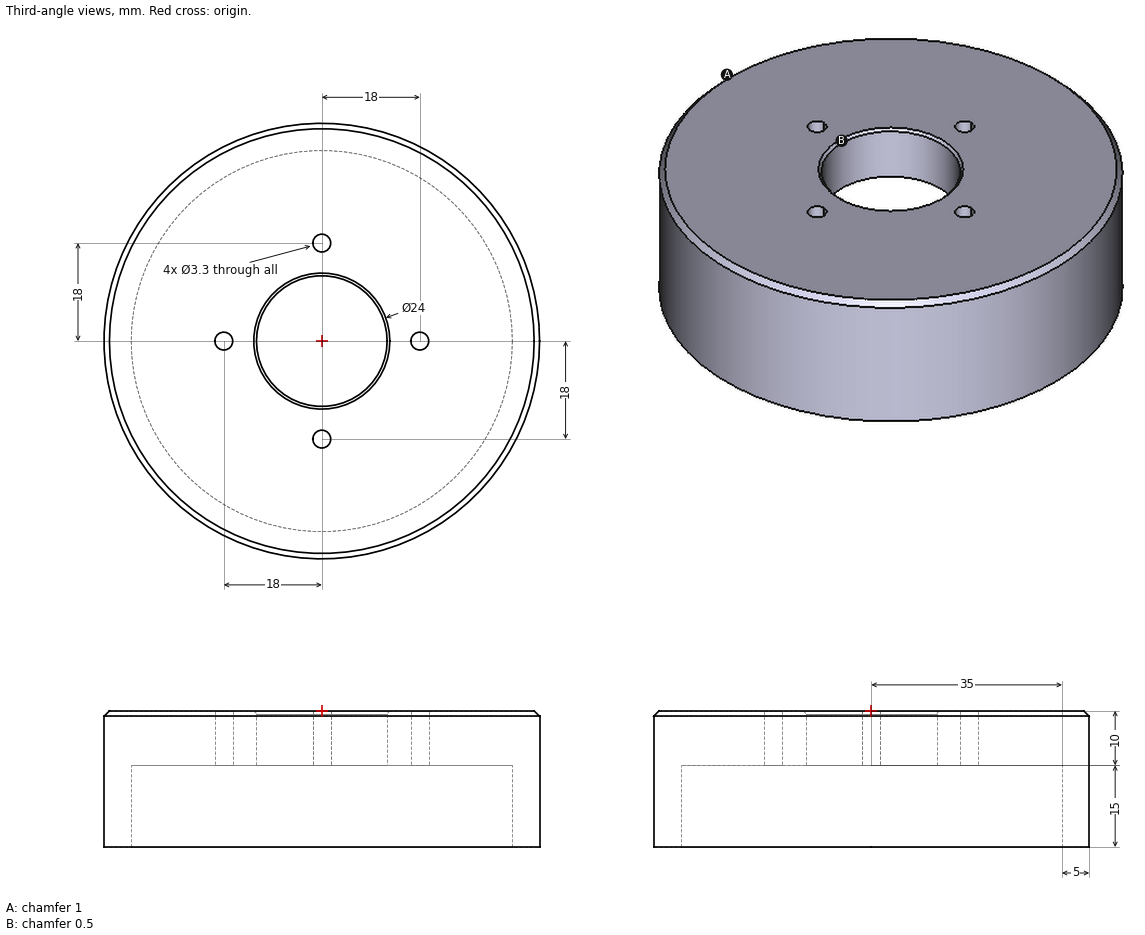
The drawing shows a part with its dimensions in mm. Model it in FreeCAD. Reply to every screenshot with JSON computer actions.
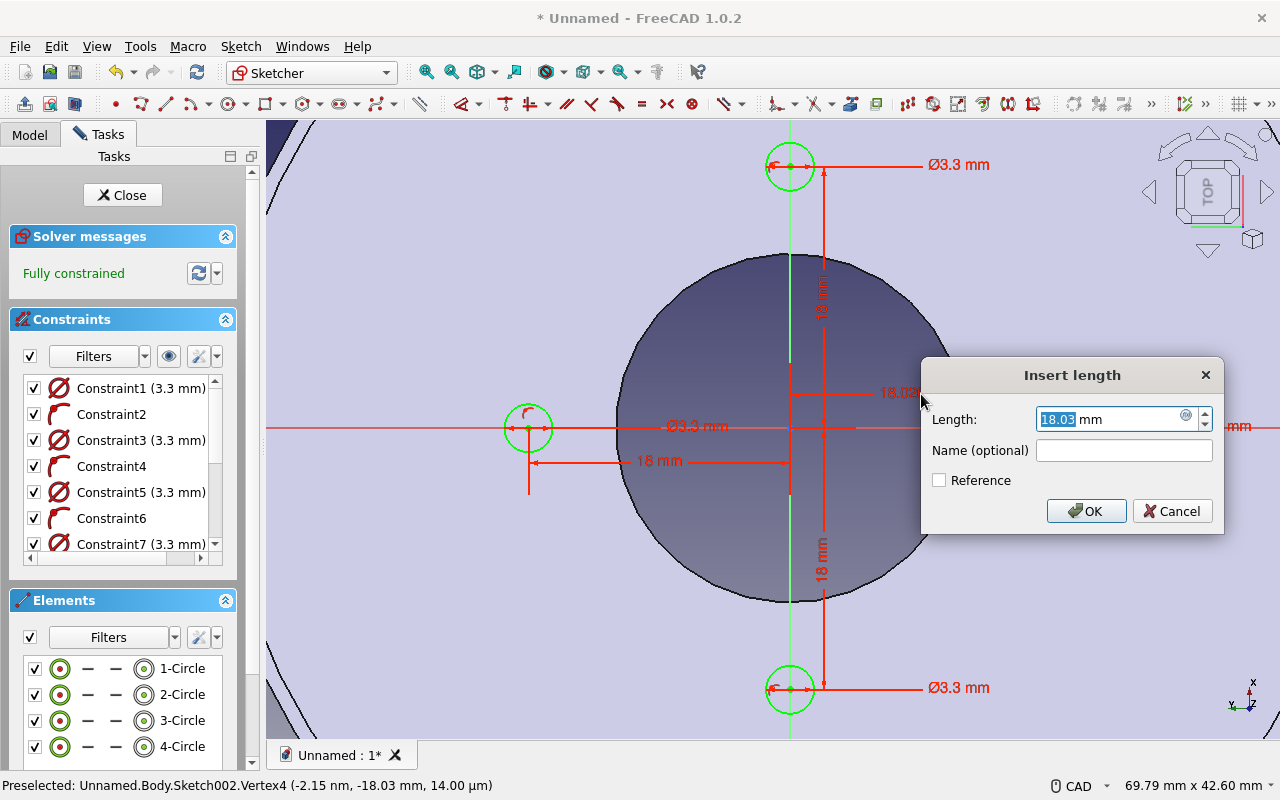
{"action": "type", "text": "18"}
{"action": "key", "text": "Return"}
{"action": "key", "text": "Escape"}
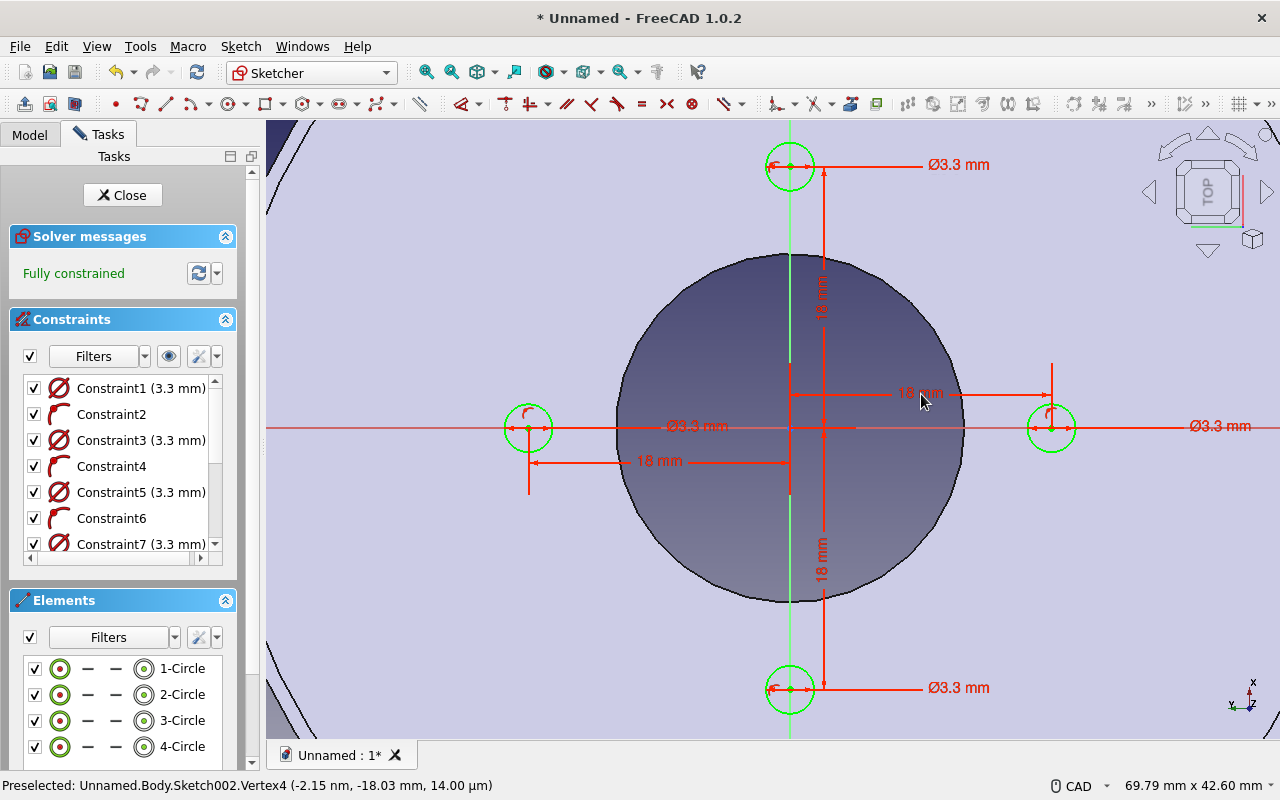
{"action": "left_click", "coordinate": [123, 195]}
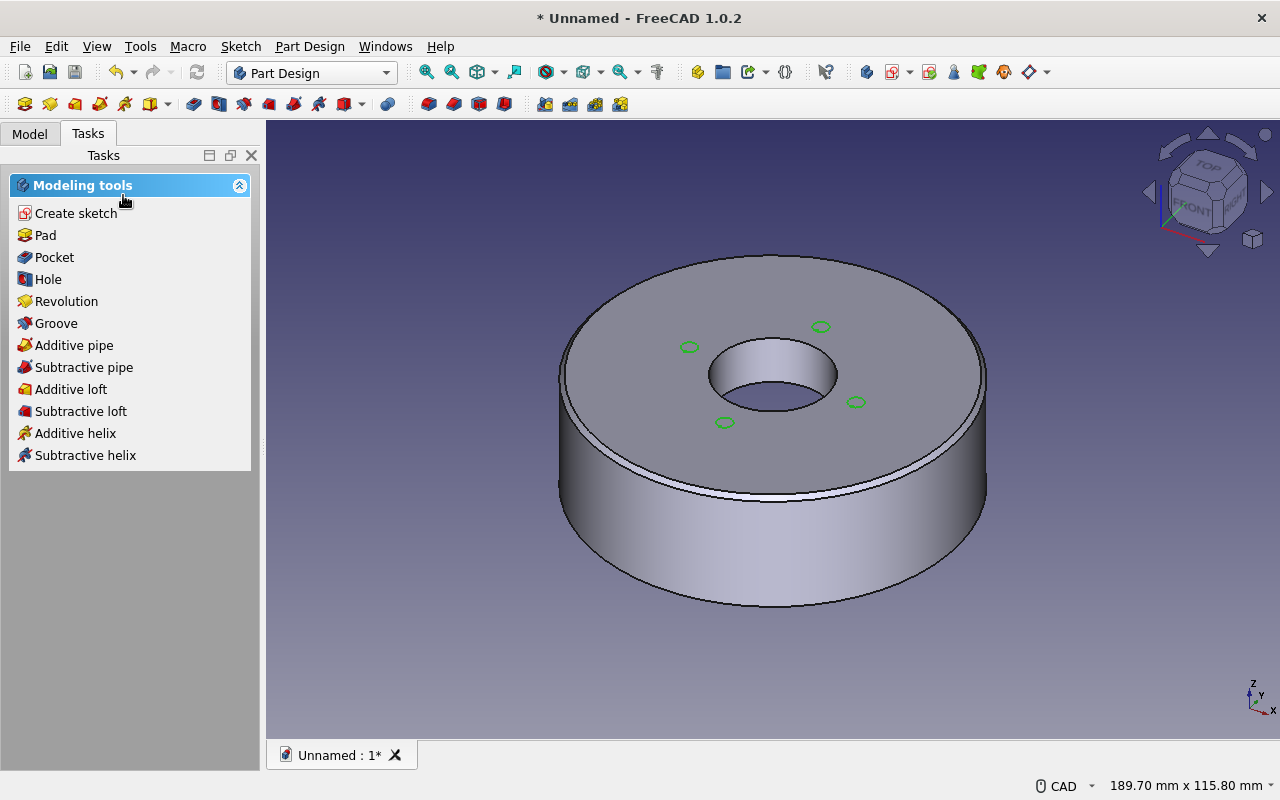
{"action": "left_click", "coordinate": [219, 104]}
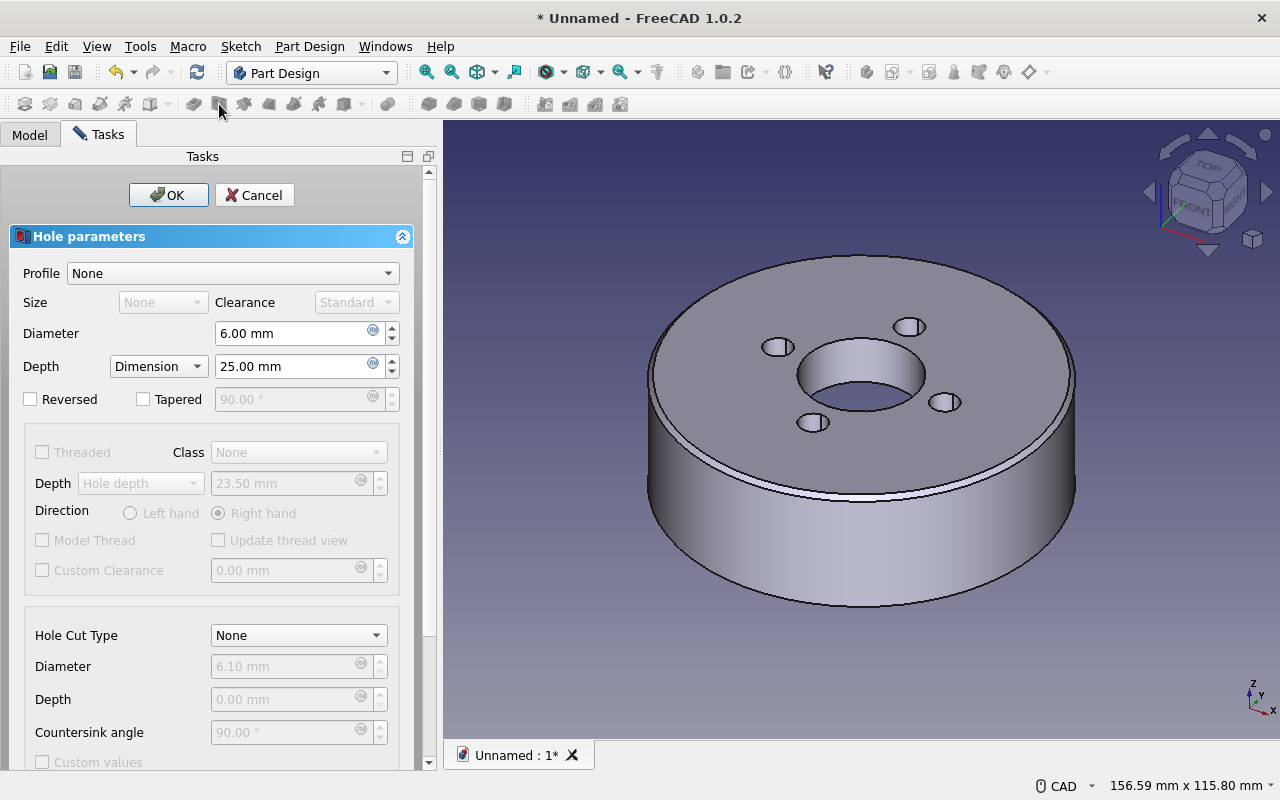
{"action": "triple_click", "coordinate": [300, 334]}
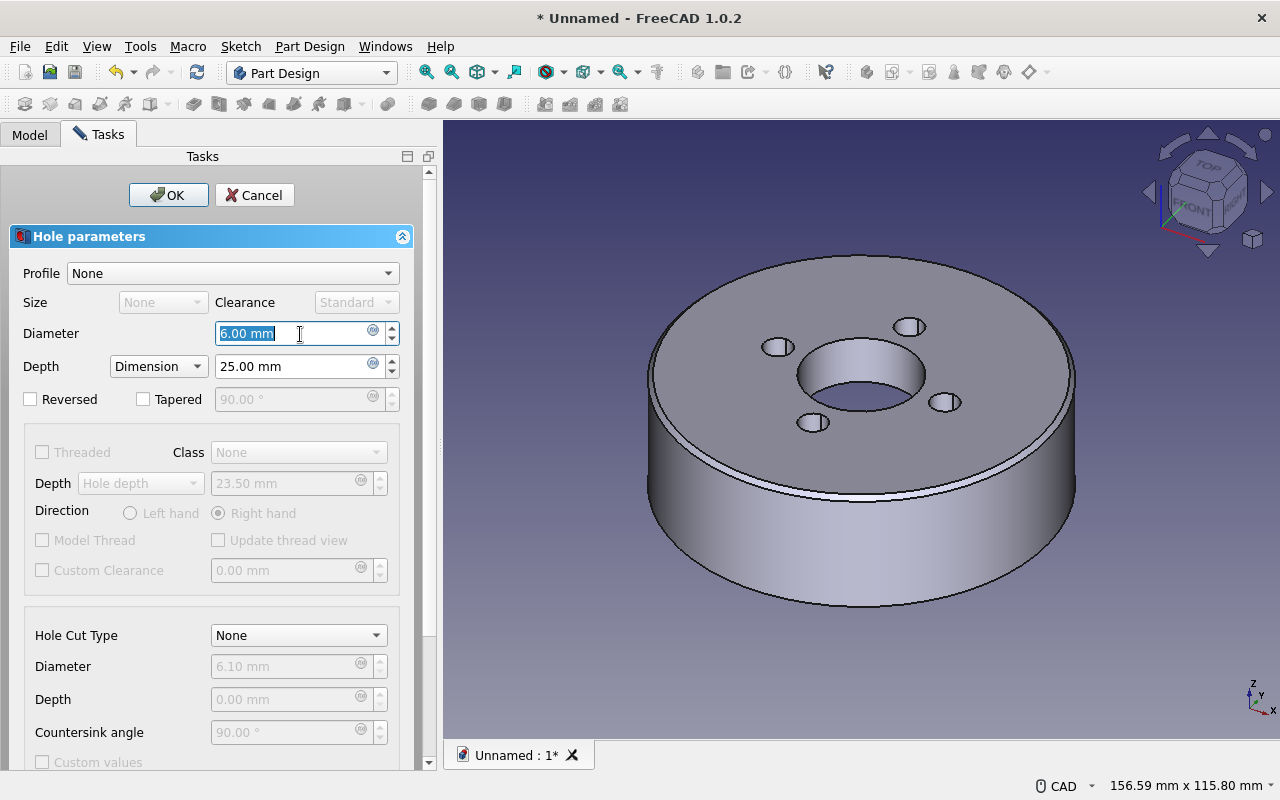
{"action": "type", "text": "3.3"}
{"action": "key", "text": "Tab"}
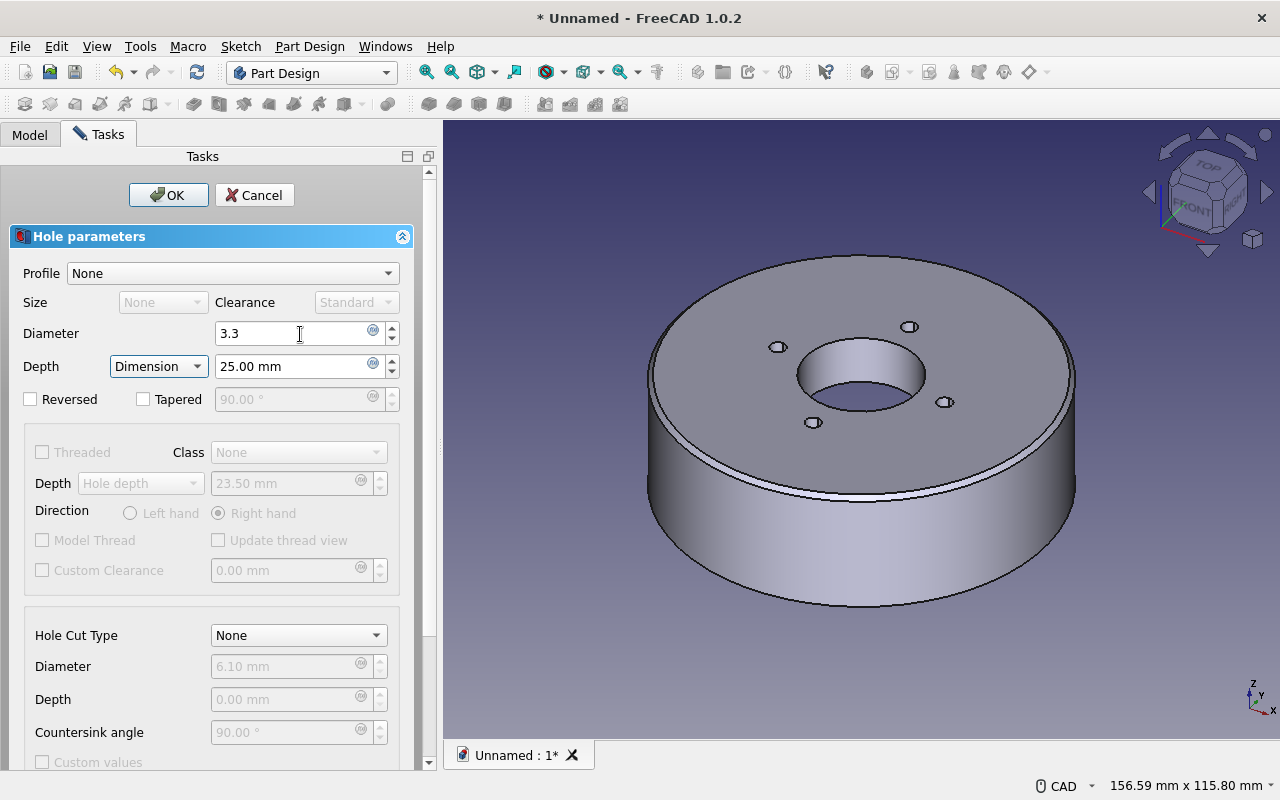
{"action": "left_click", "coordinate": [160, 366]}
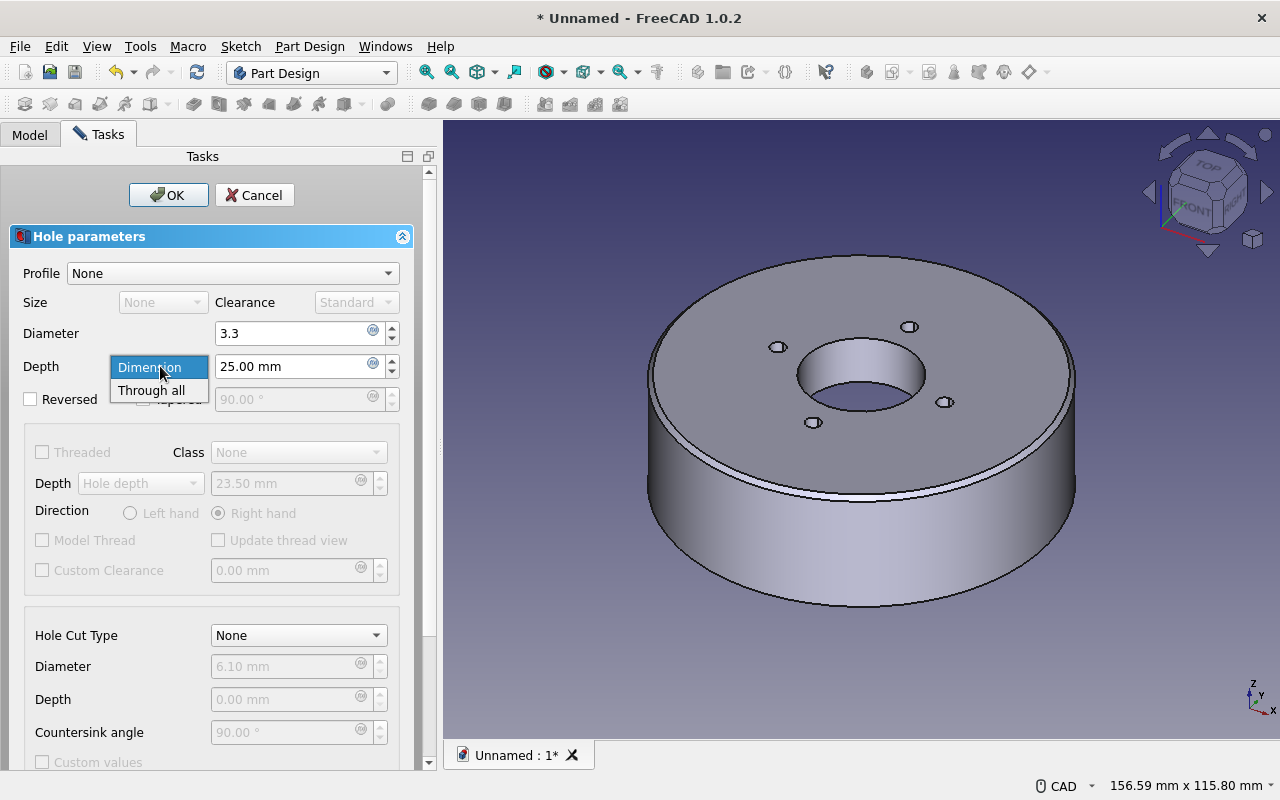
{"action": "left_click", "coordinate": [158, 390]}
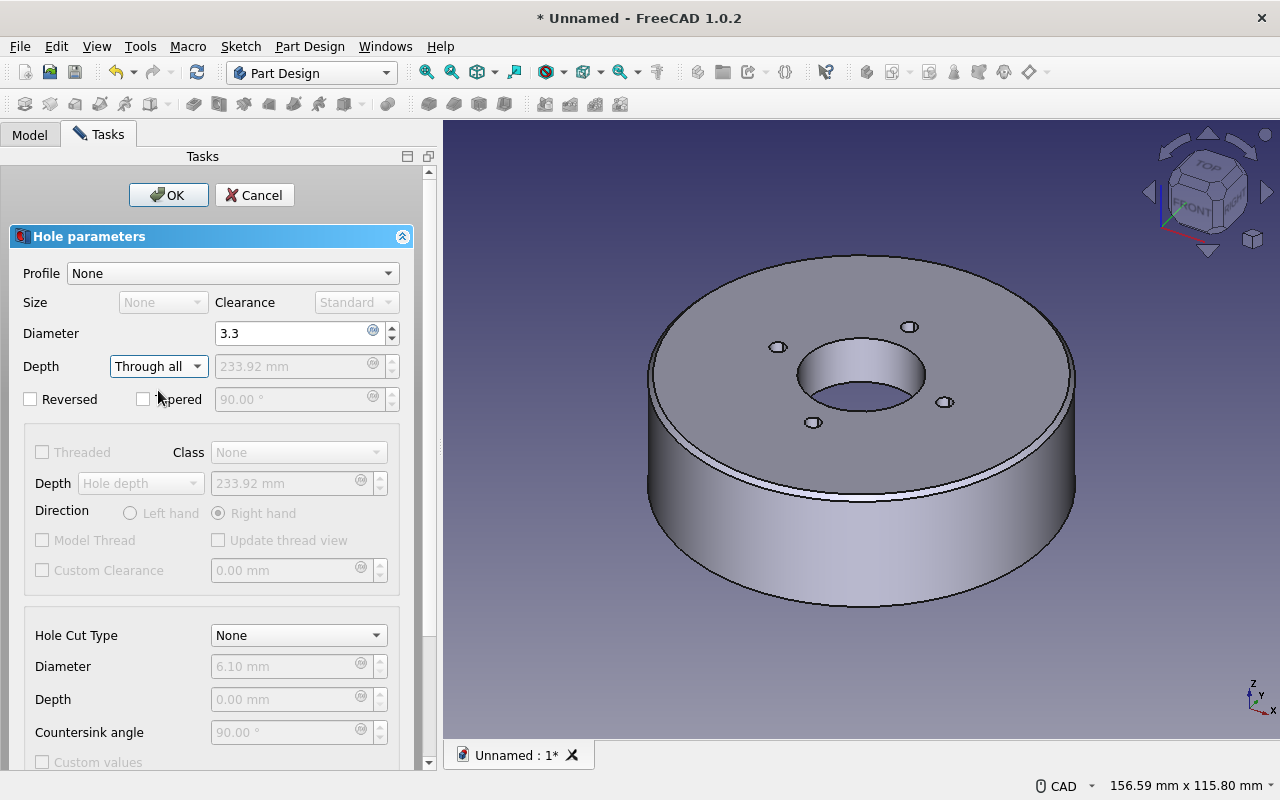
{"action": "left_click", "coordinate": [169, 195]}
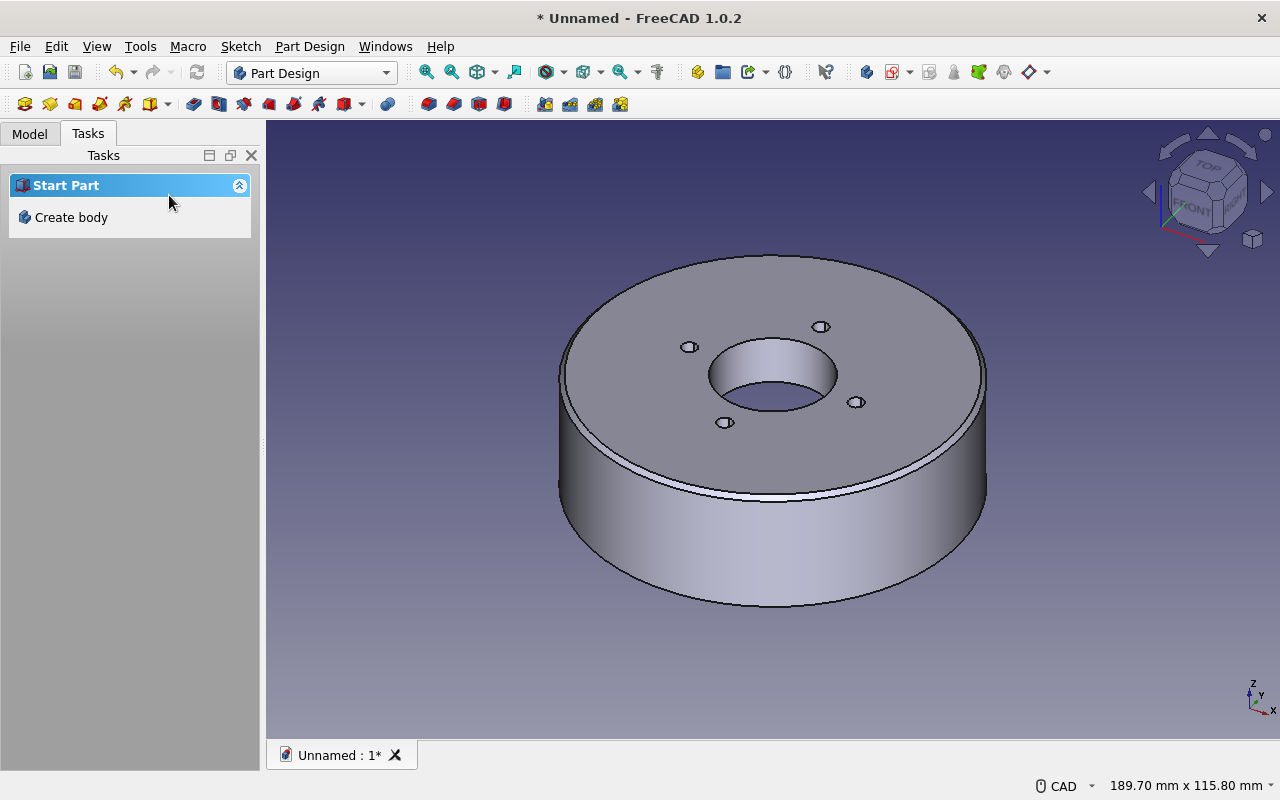
{"action": "left_click", "coordinate": [805, 342]}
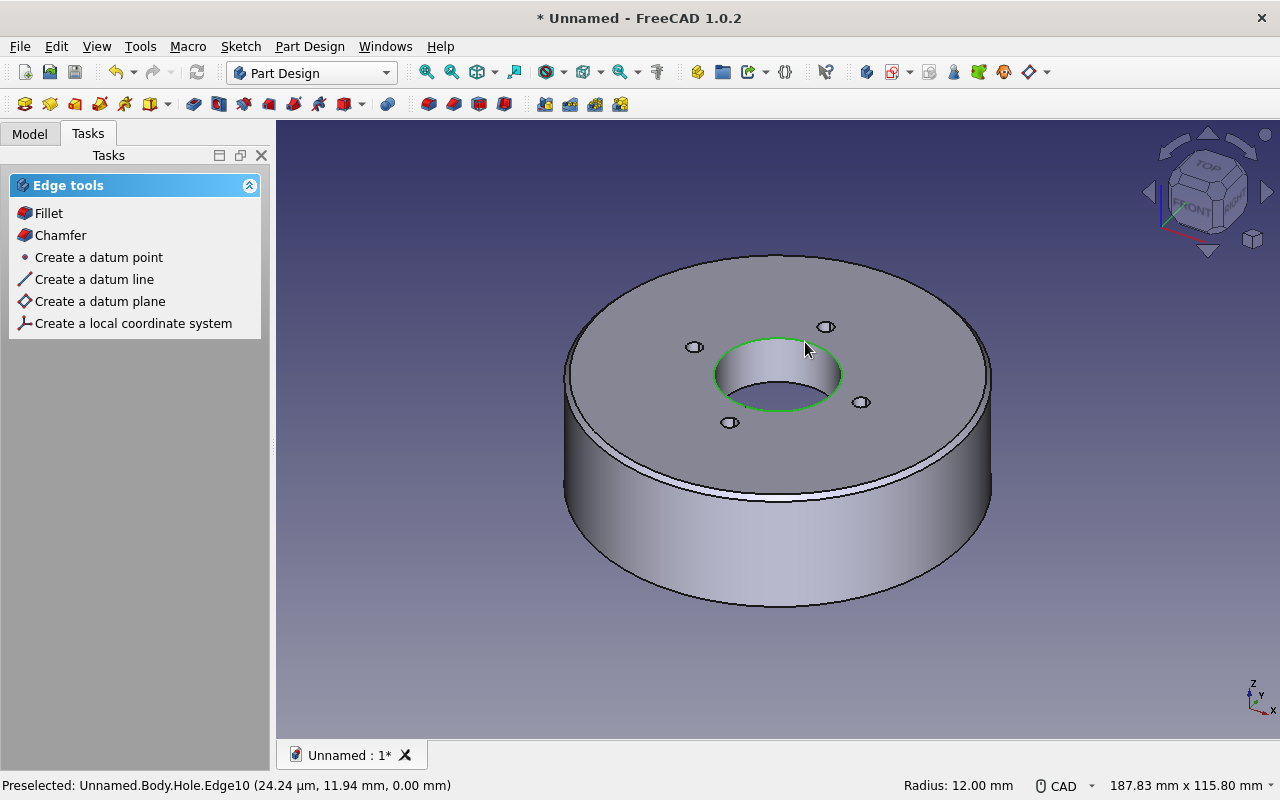
{"action": "left_click", "coordinate": [454, 104]}